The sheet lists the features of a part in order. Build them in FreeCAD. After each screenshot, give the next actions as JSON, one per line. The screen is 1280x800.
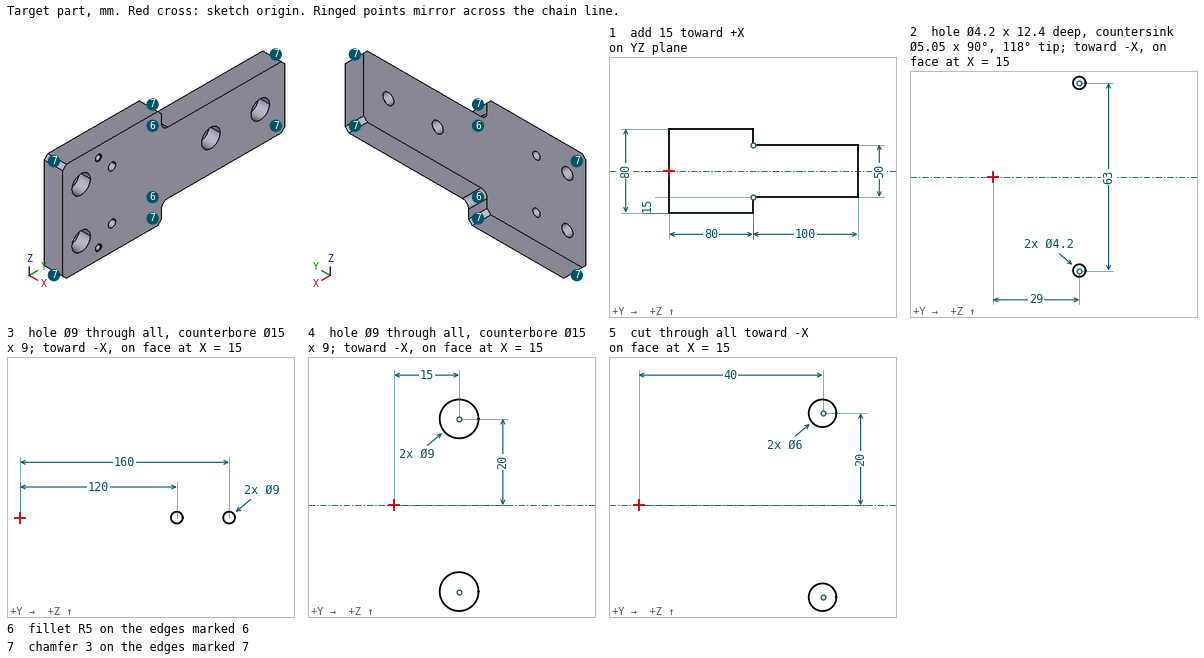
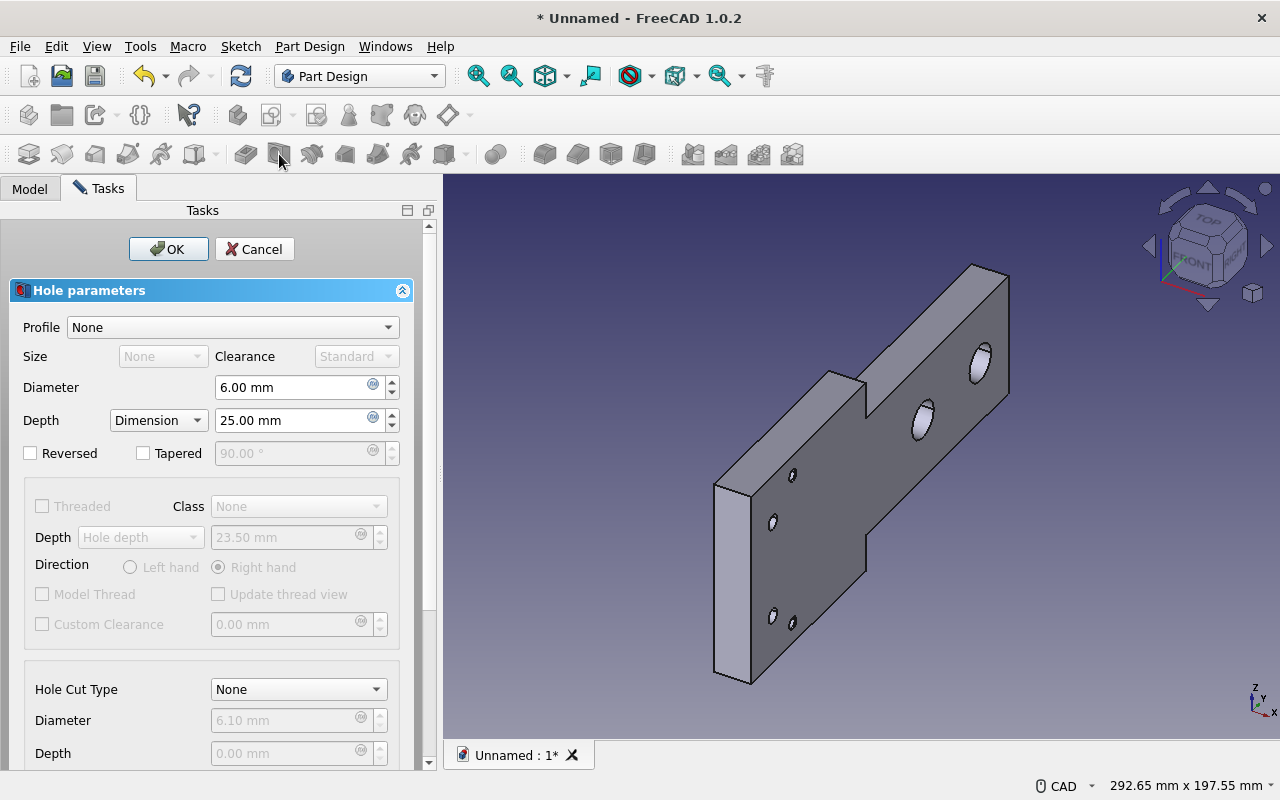
{"action": "triple_click", "coordinate": [300, 388]}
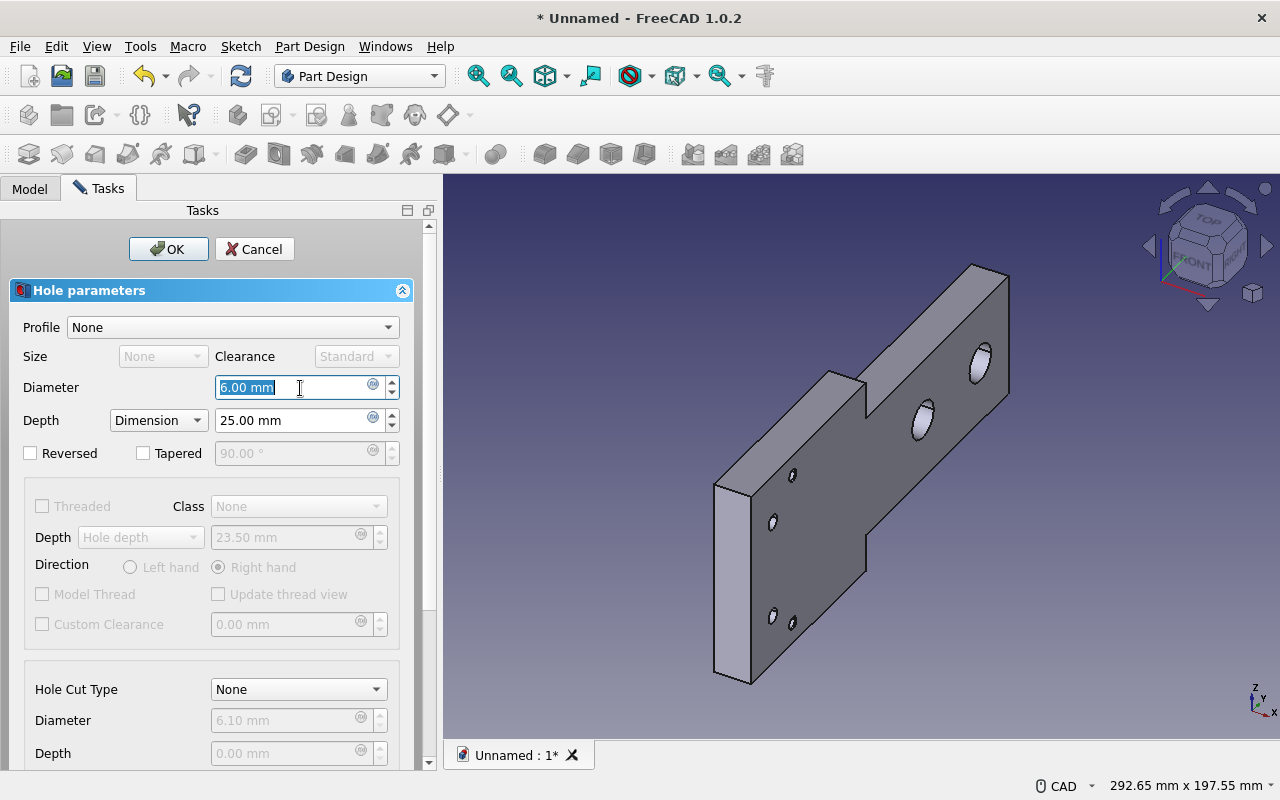
{"action": "type", "text": "9"}
{"action": "key", "text": "Tab"}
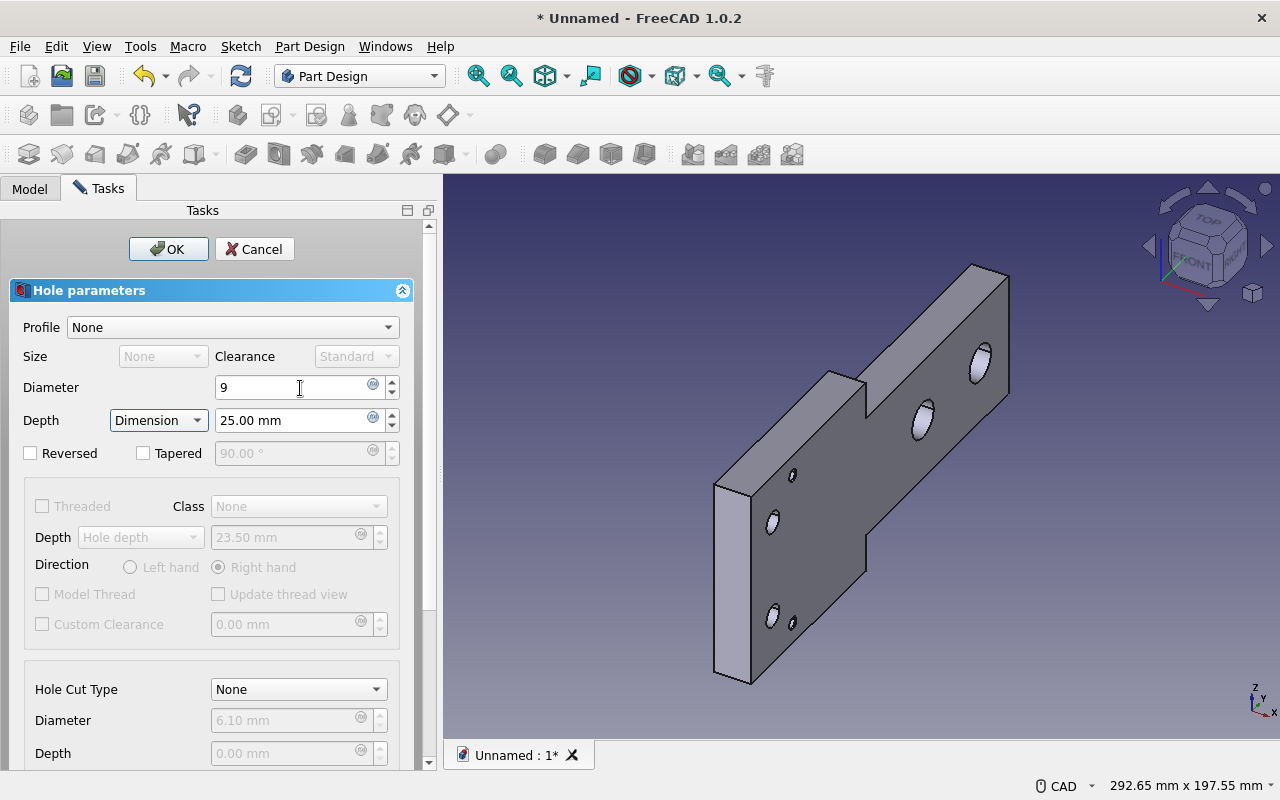
{"action": "left_click", "coordinate": [160, 420]}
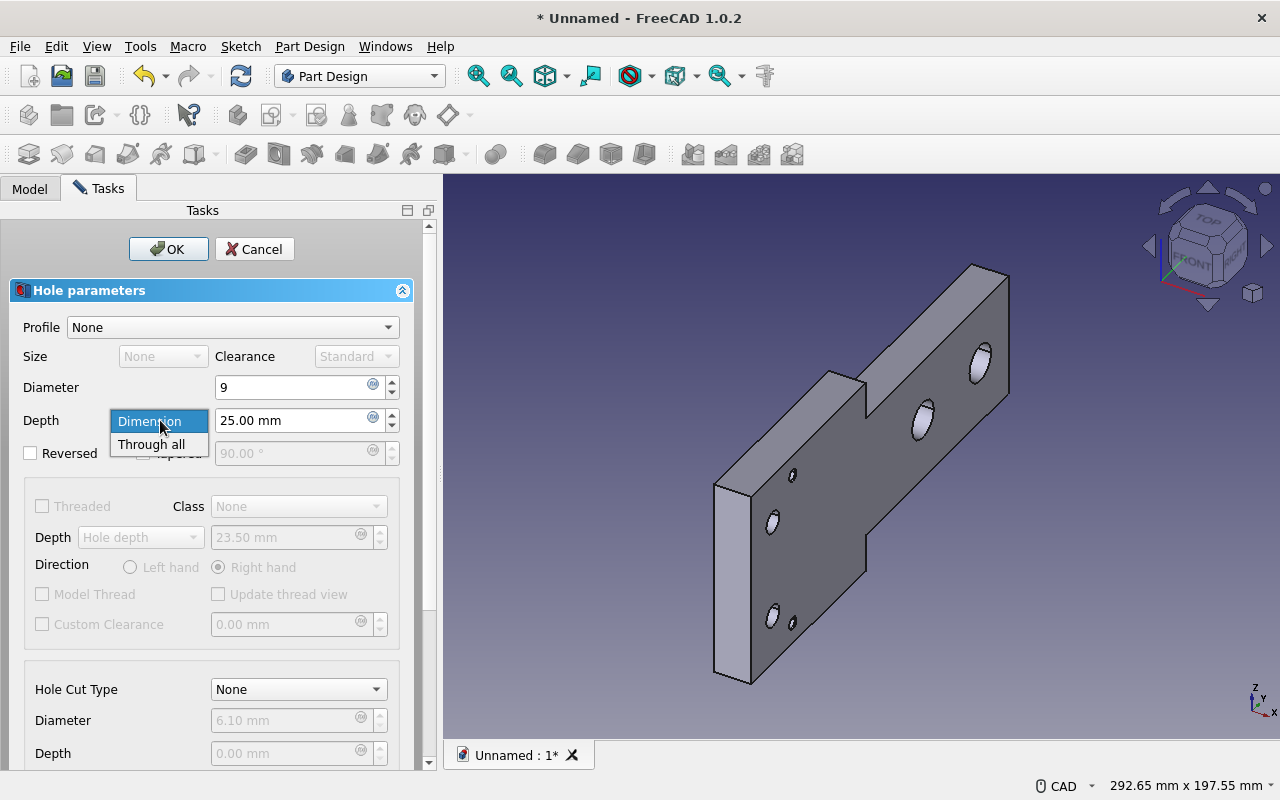
{"action": "left_click", "coordinate": [158, 444]}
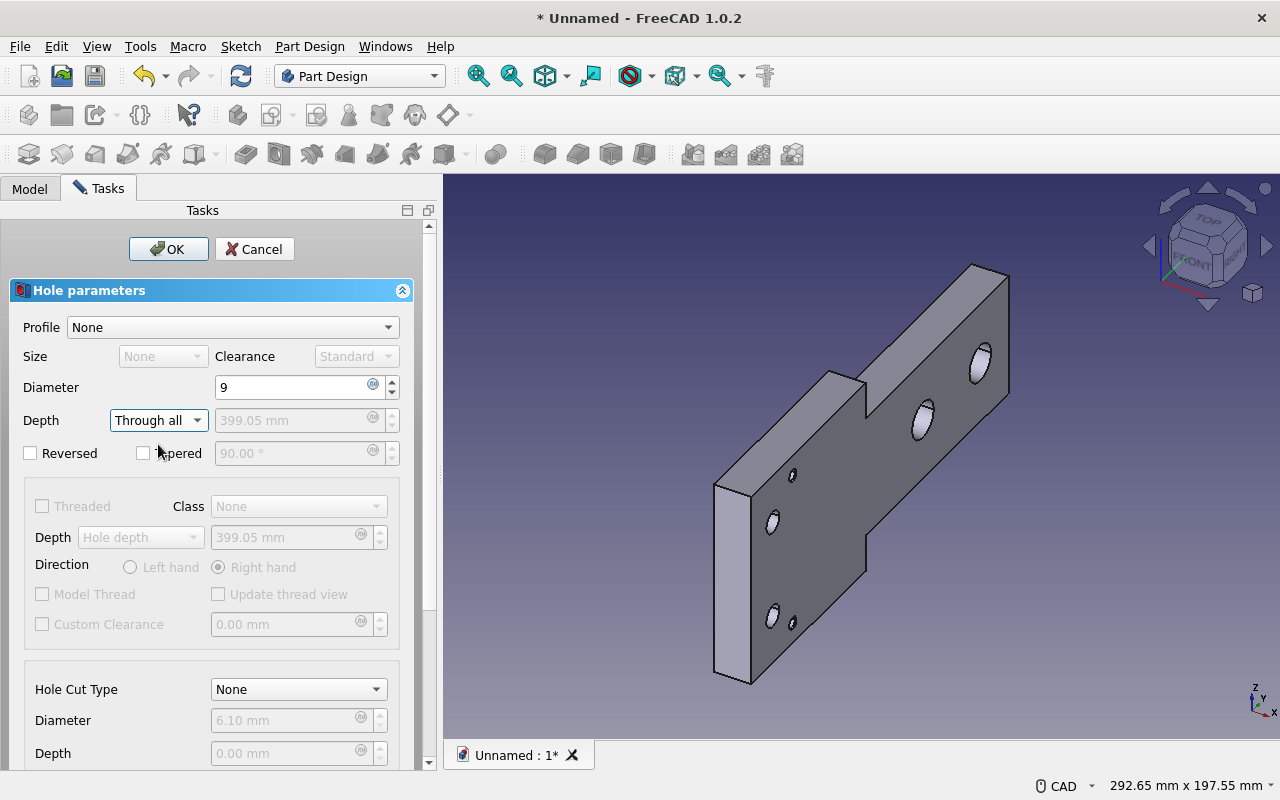
{"action": "left_click", "coordinate": [300, 690]}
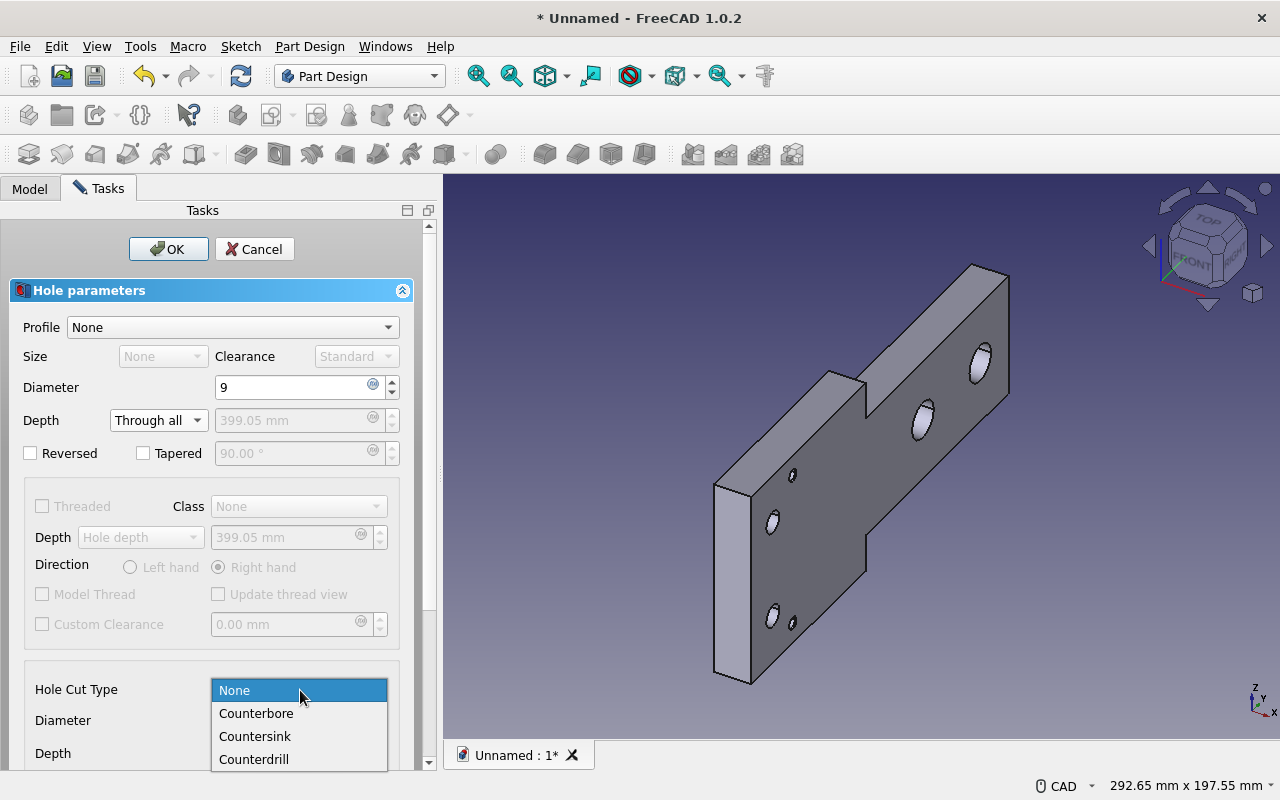
{"action": "left_click", "coordinate": [298, 714]}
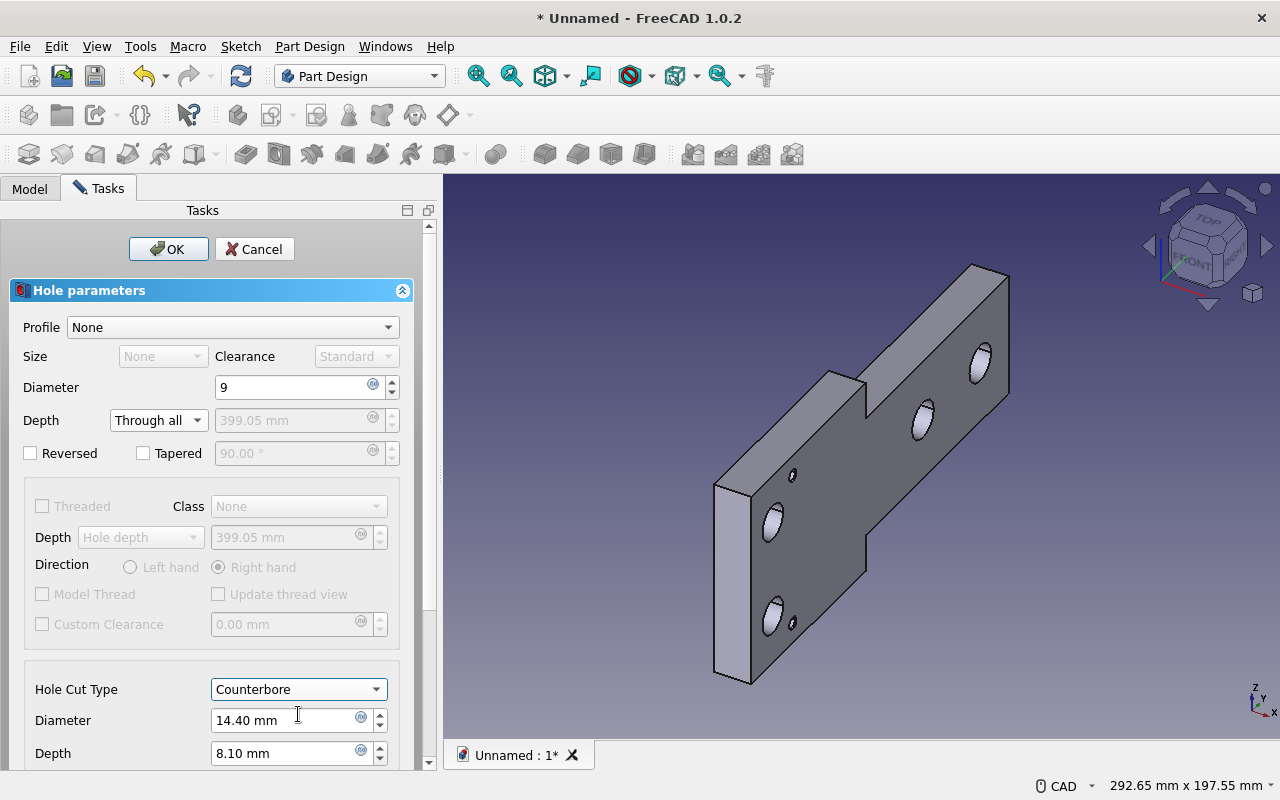
{"action": "triple_click", "coordinate": [292, 720]}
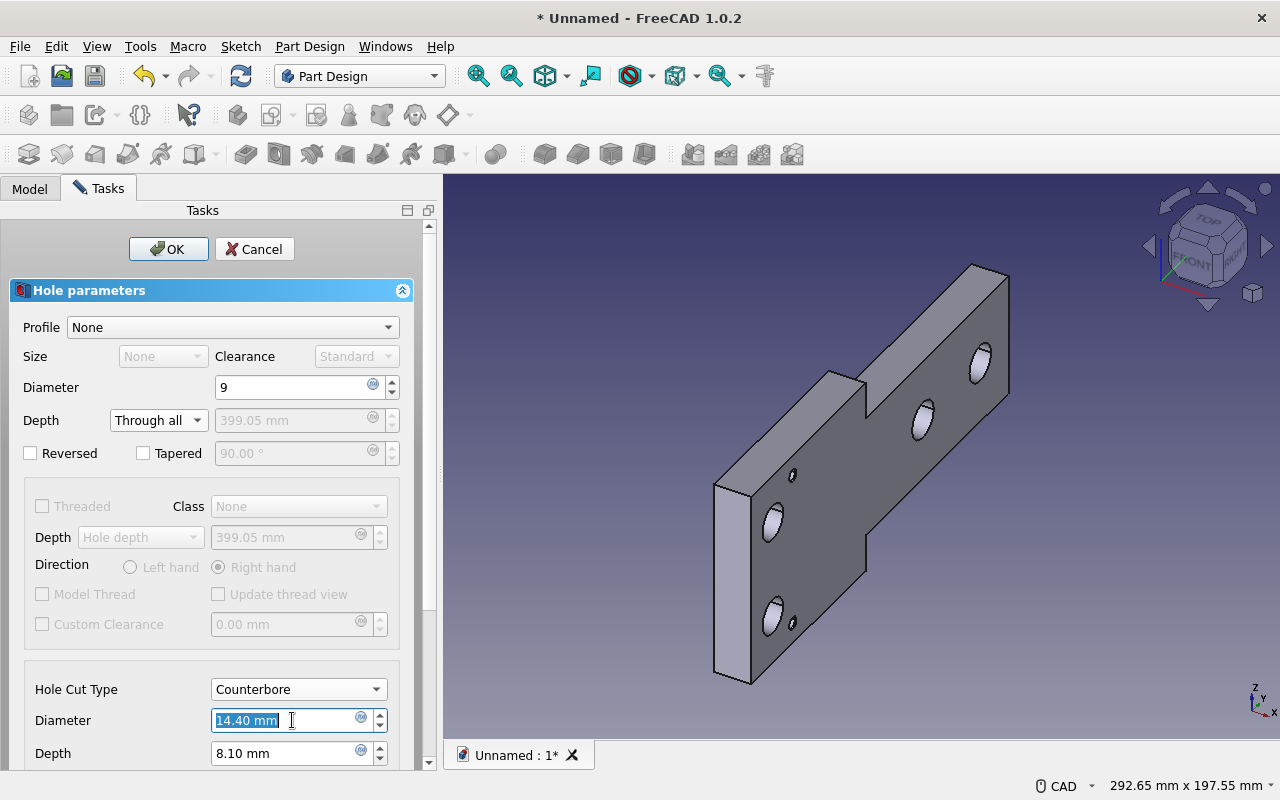
{"action": "type", "text": "15"}
{"action": "key", "text": "Tab"}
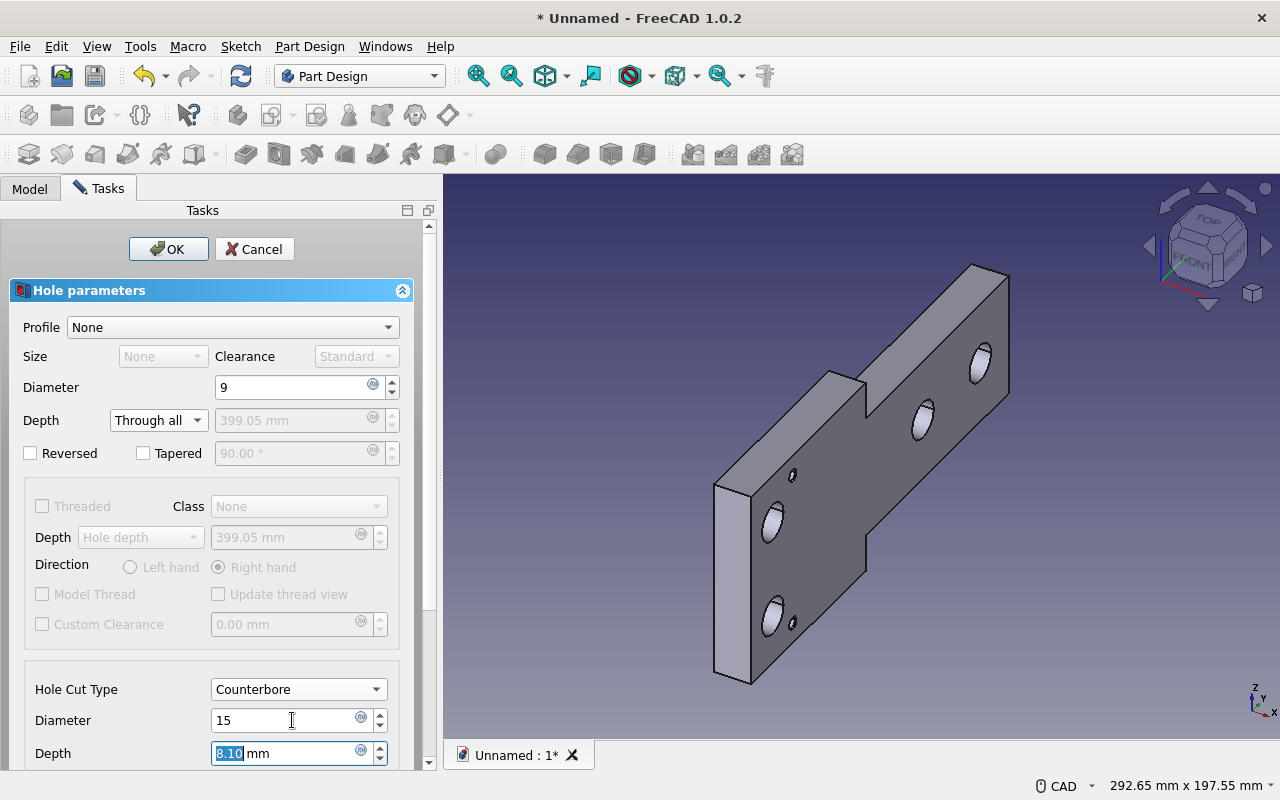
{"action": "type", "text": "9"}
{"action": "key", "text": "Tab"}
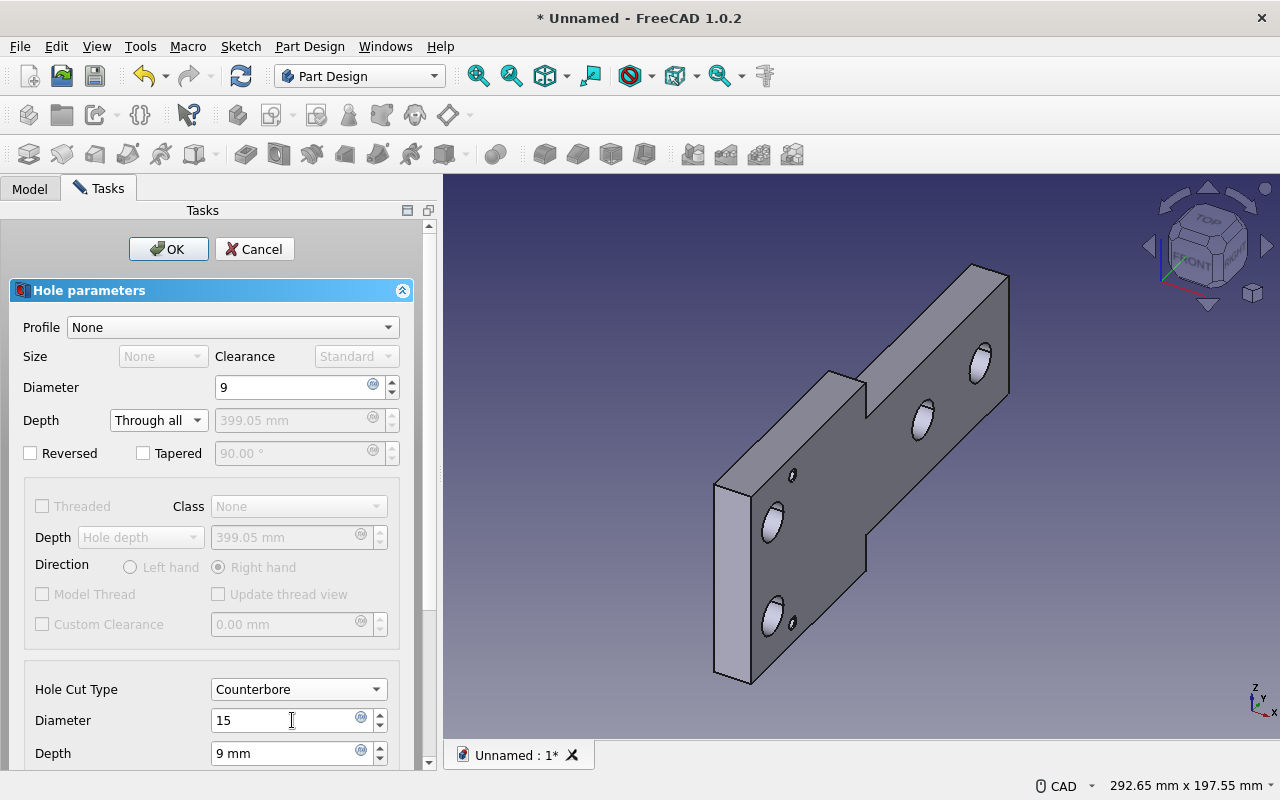
{"action": "left_click", "coordinate": [169, 249]}